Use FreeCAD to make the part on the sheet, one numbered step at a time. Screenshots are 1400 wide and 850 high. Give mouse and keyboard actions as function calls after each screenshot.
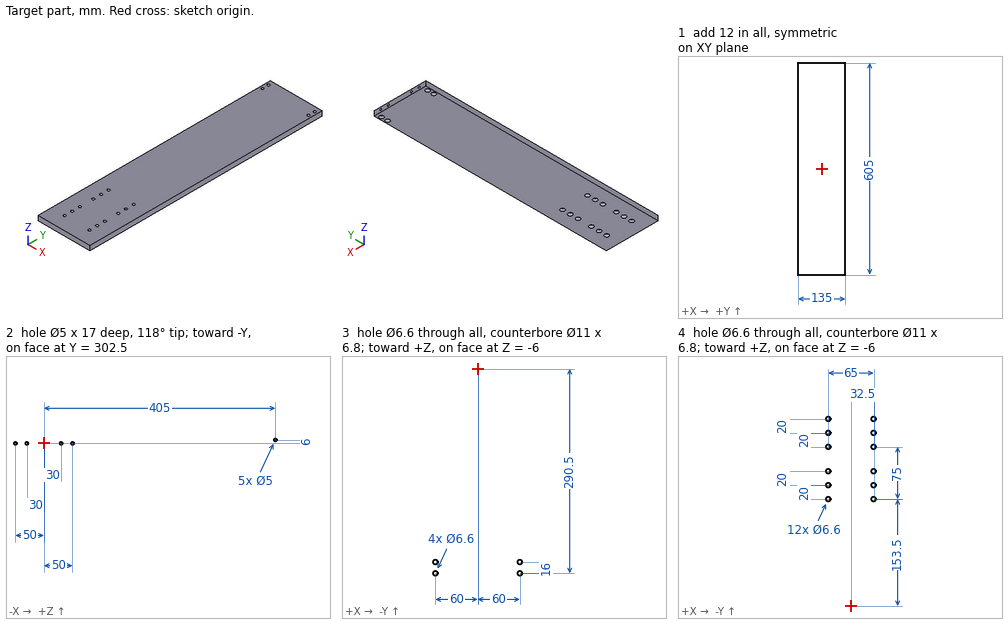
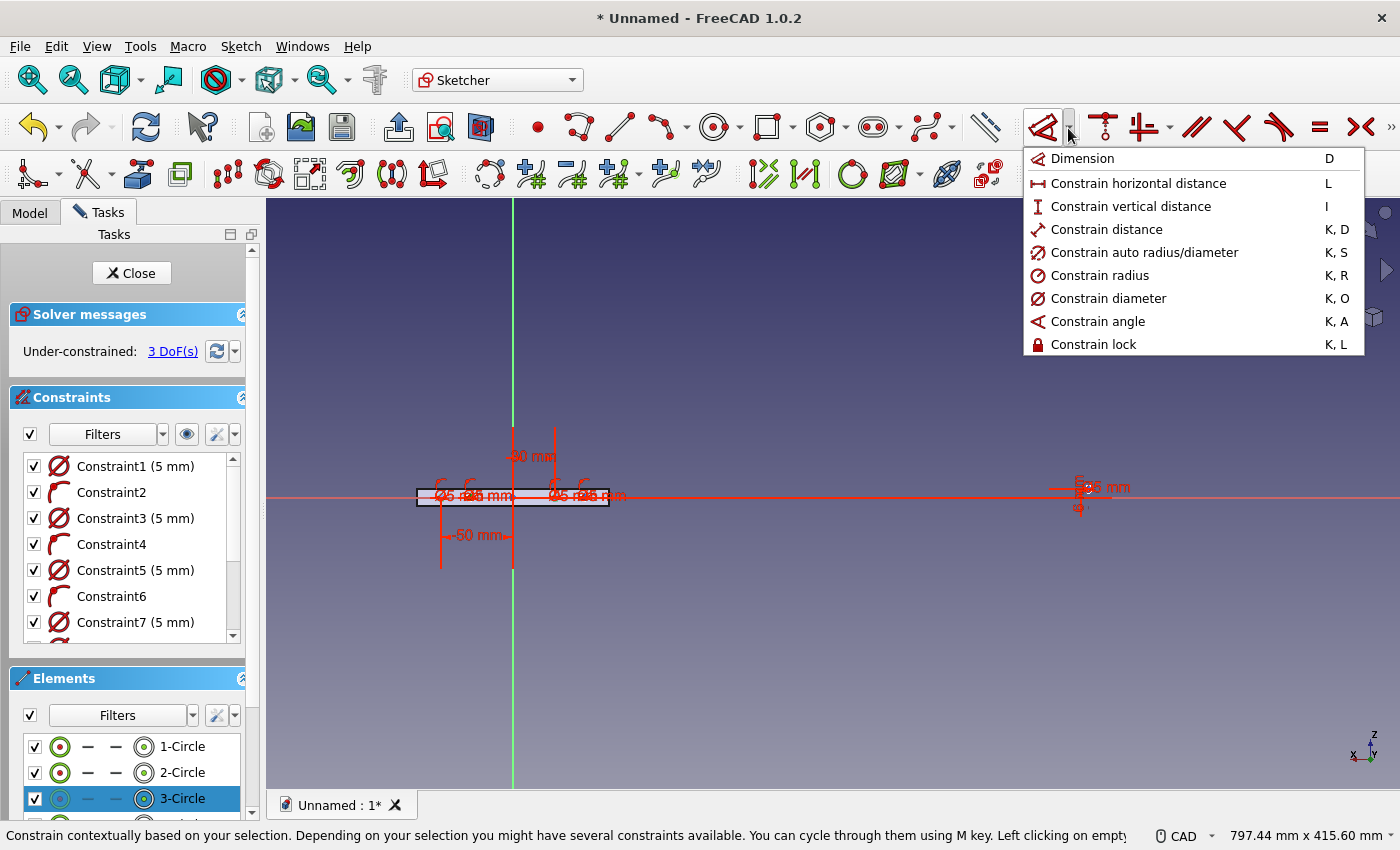
click(1194, 184)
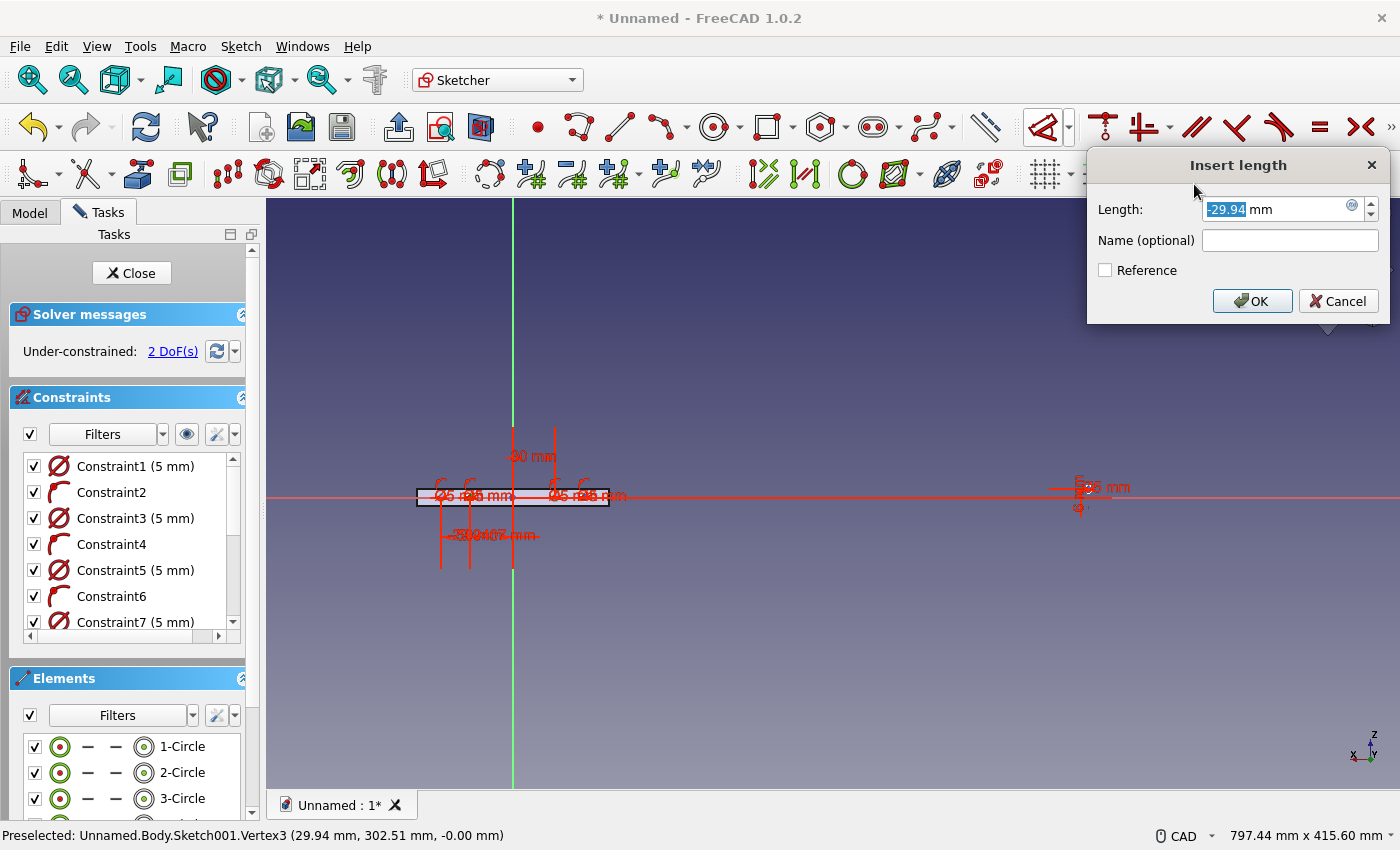
text(-30)
key(Return)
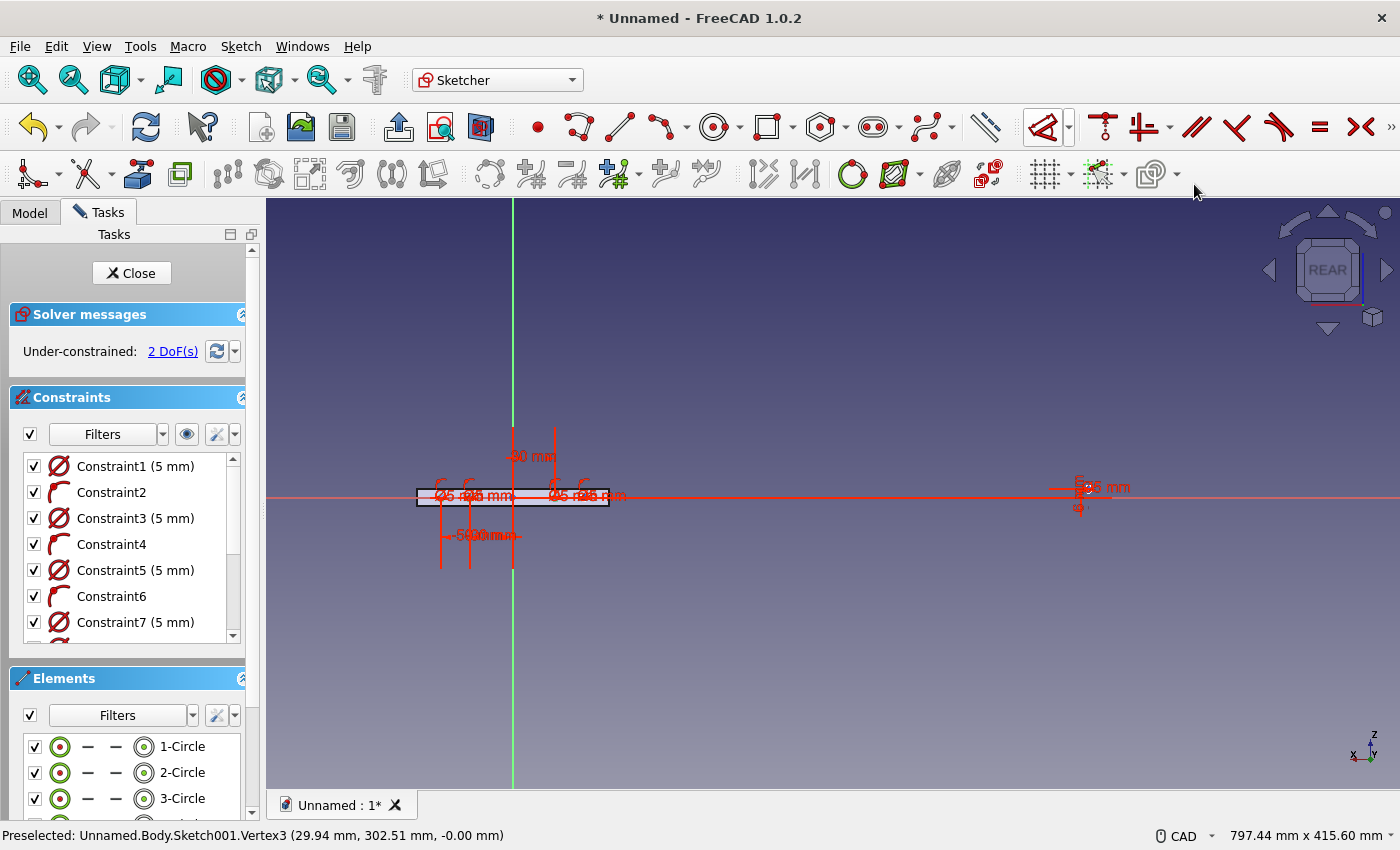
click(584, 498)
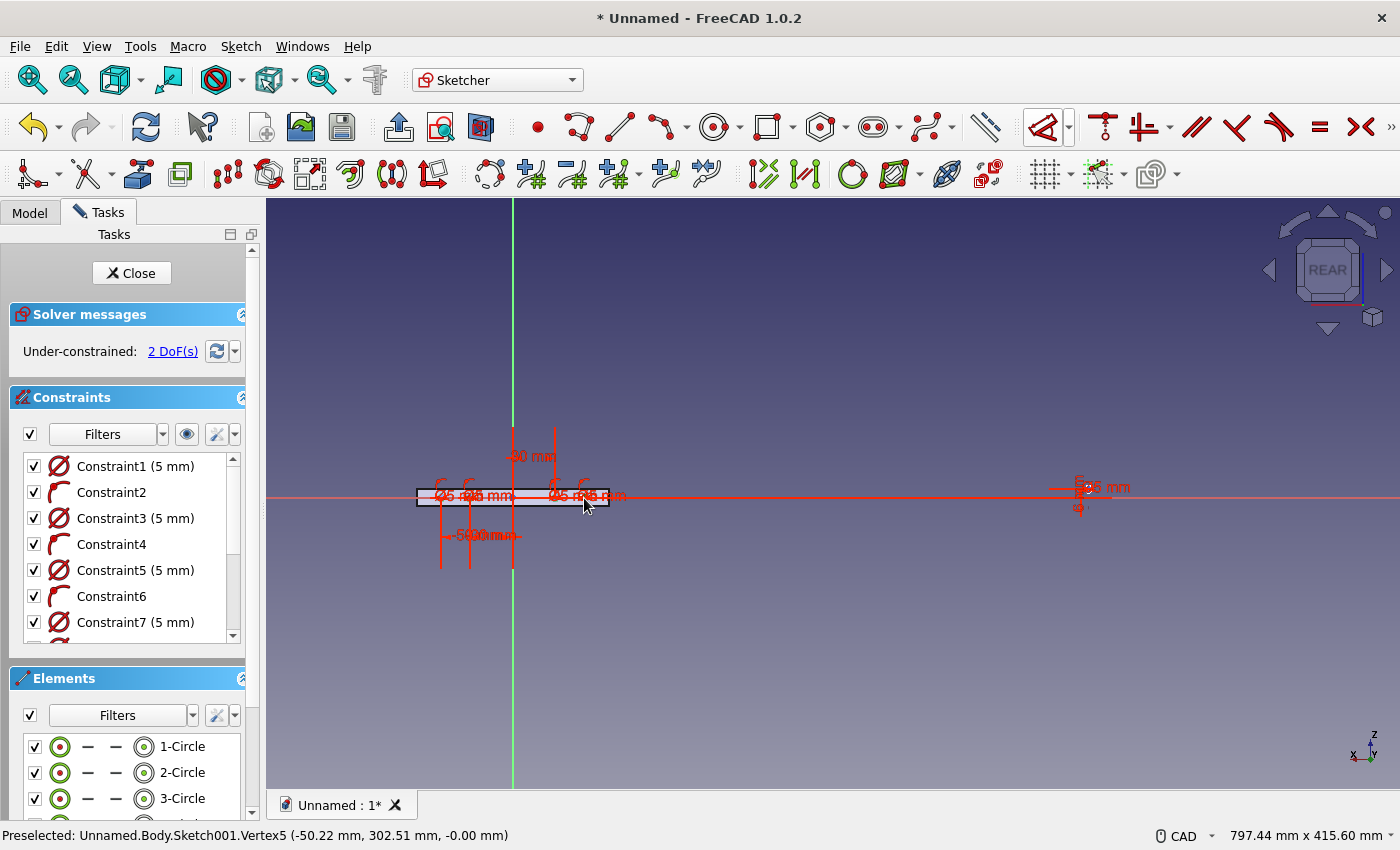
click(1068, 128)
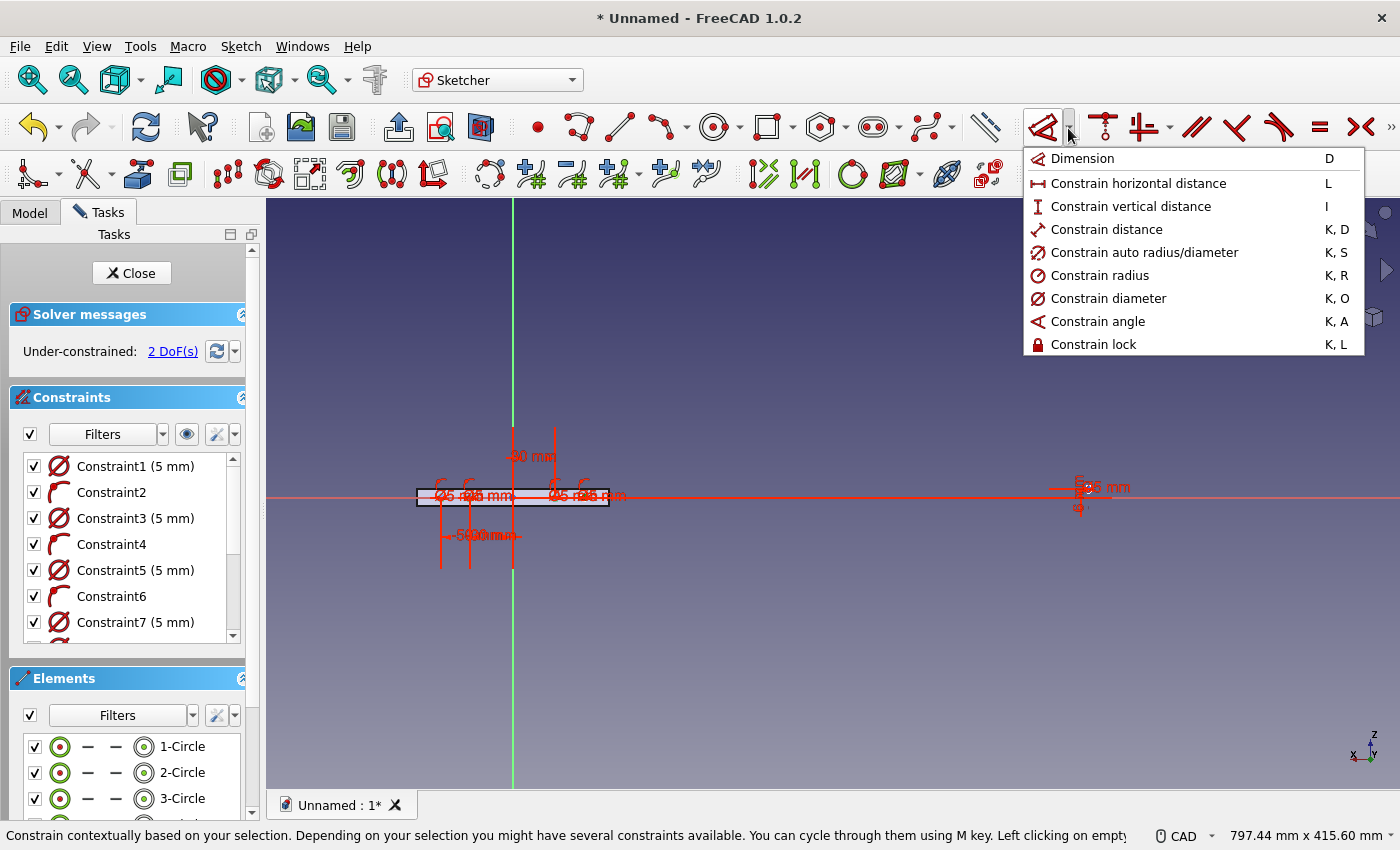
click(1194, 184)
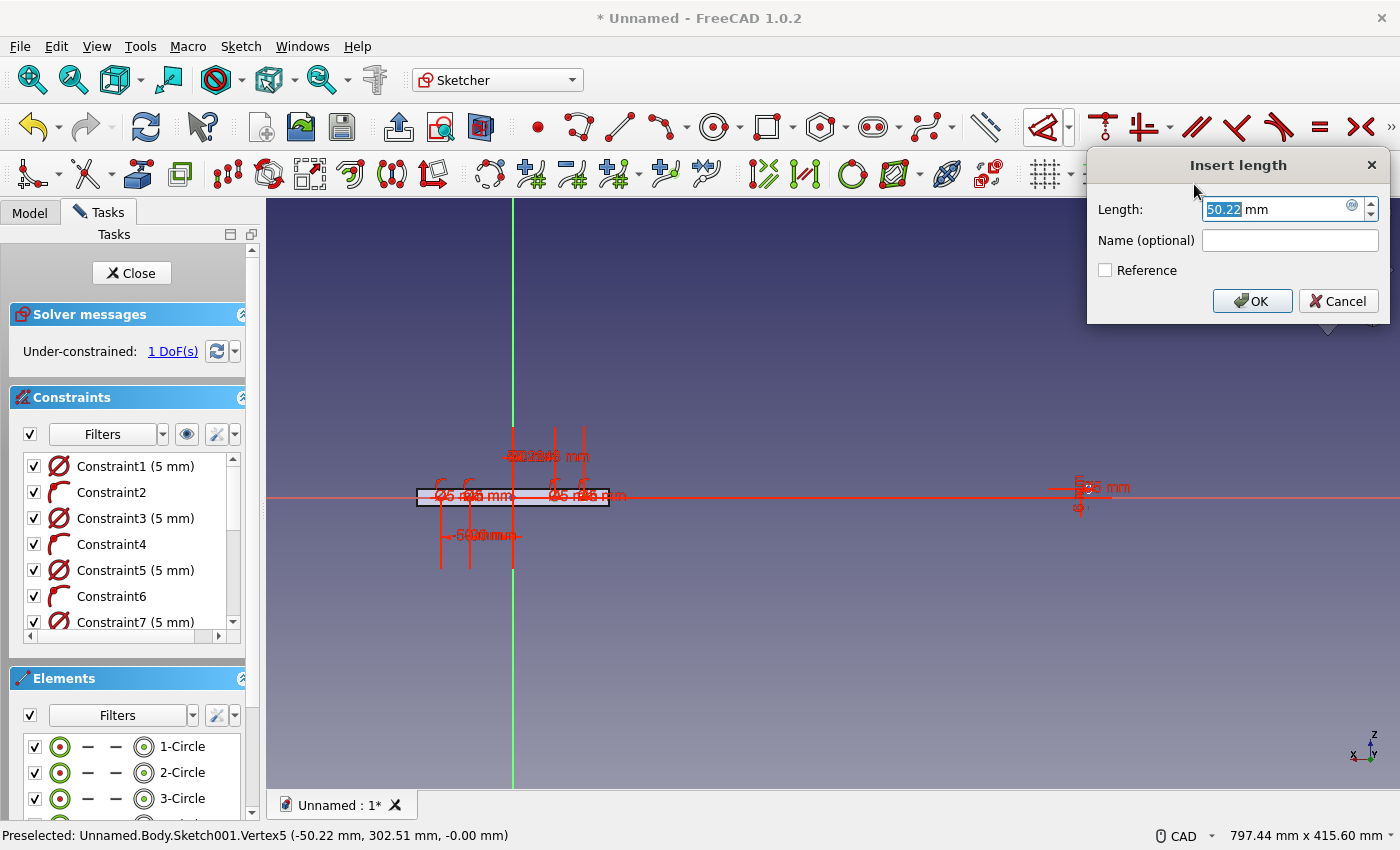
text(50)
key(Return)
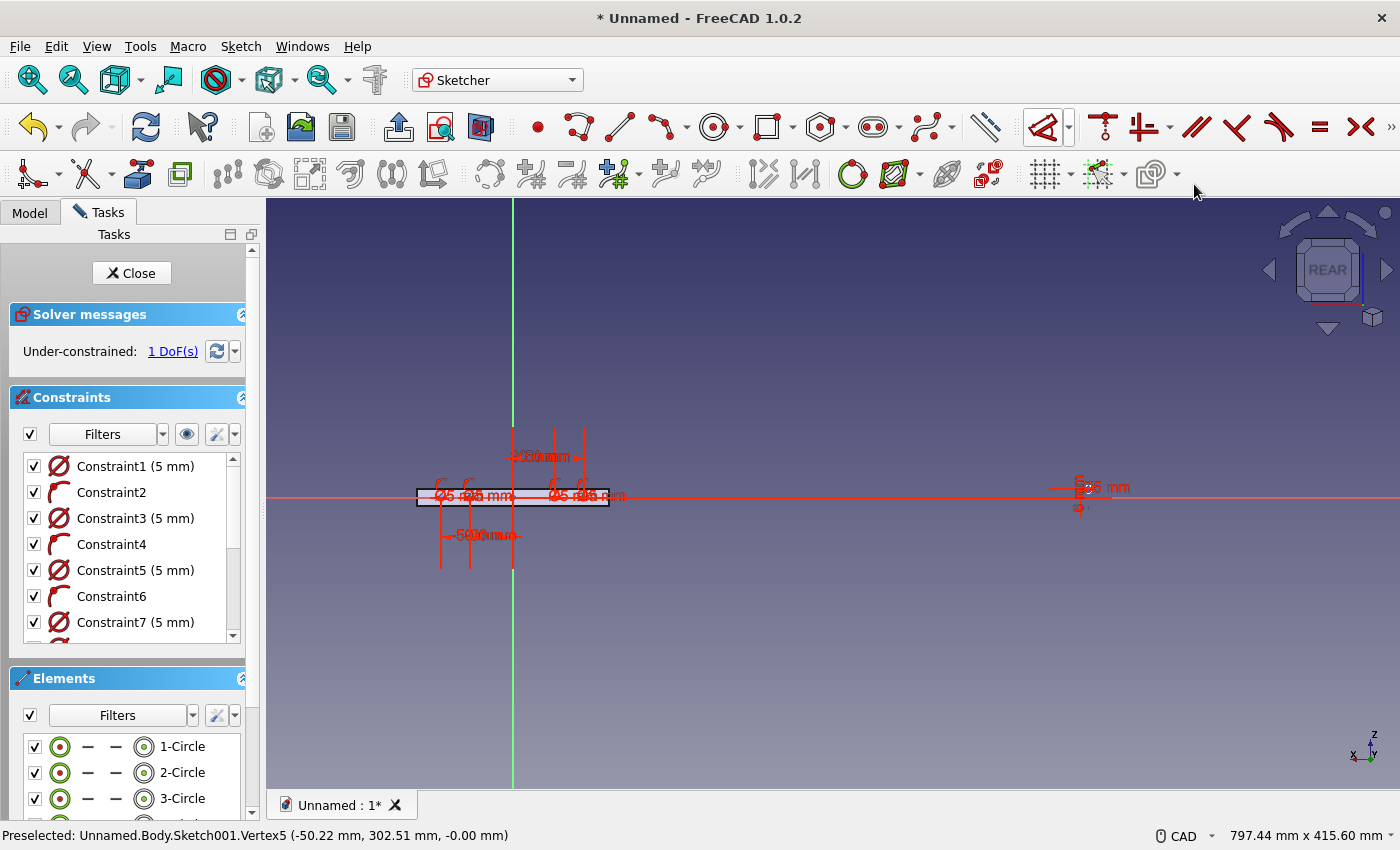
click(1089, 489)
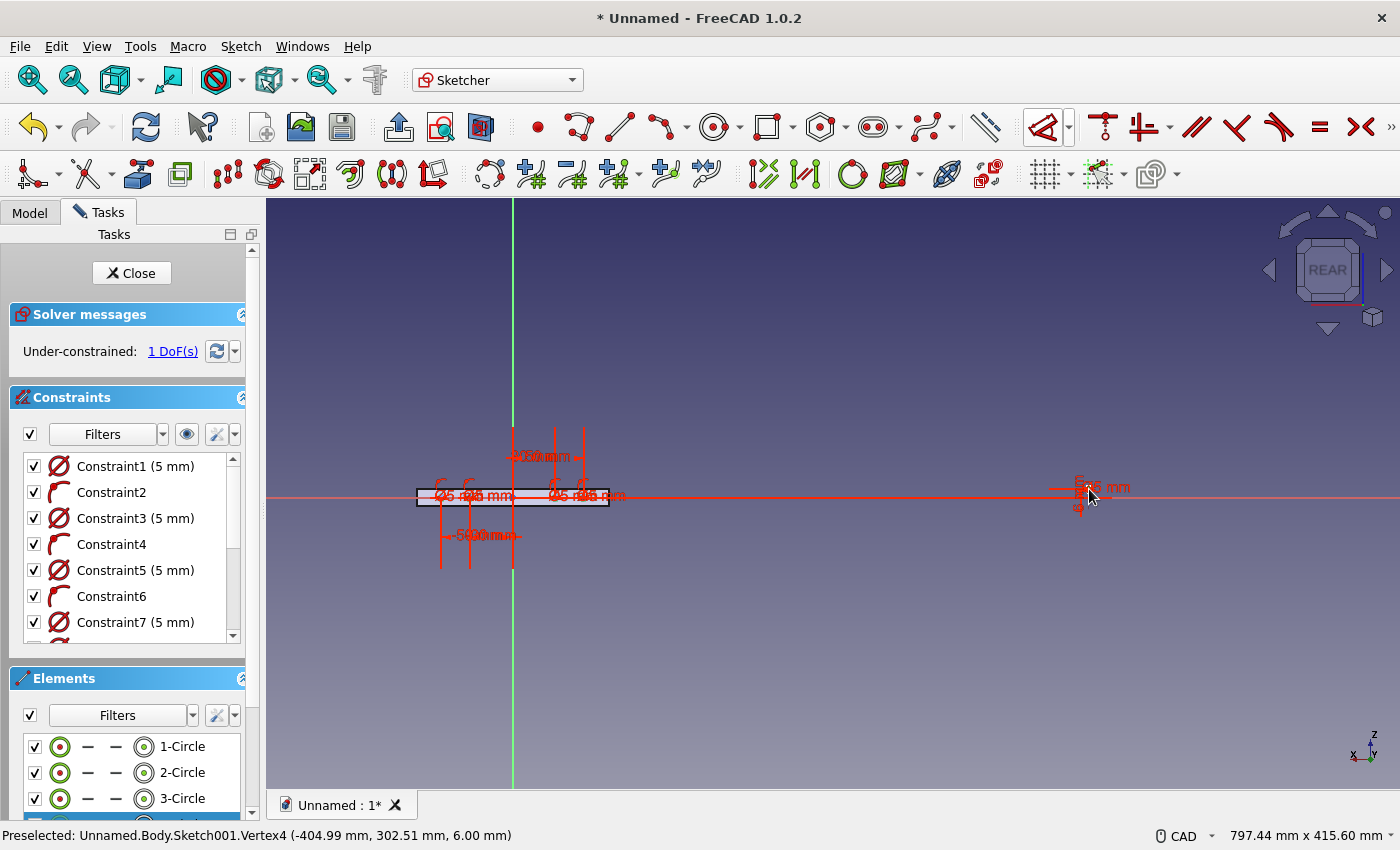
key(l)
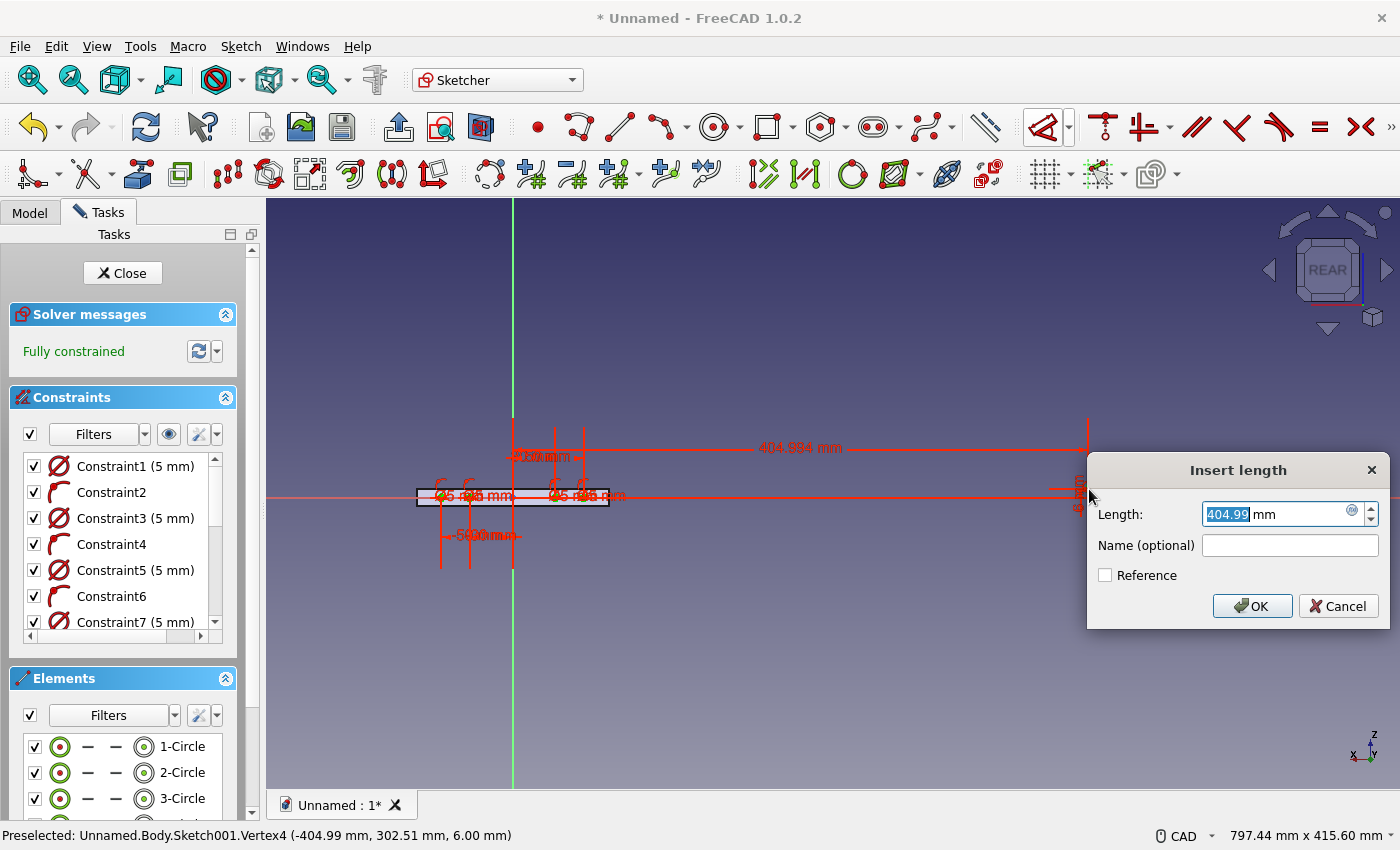
text(405)
key(Return)